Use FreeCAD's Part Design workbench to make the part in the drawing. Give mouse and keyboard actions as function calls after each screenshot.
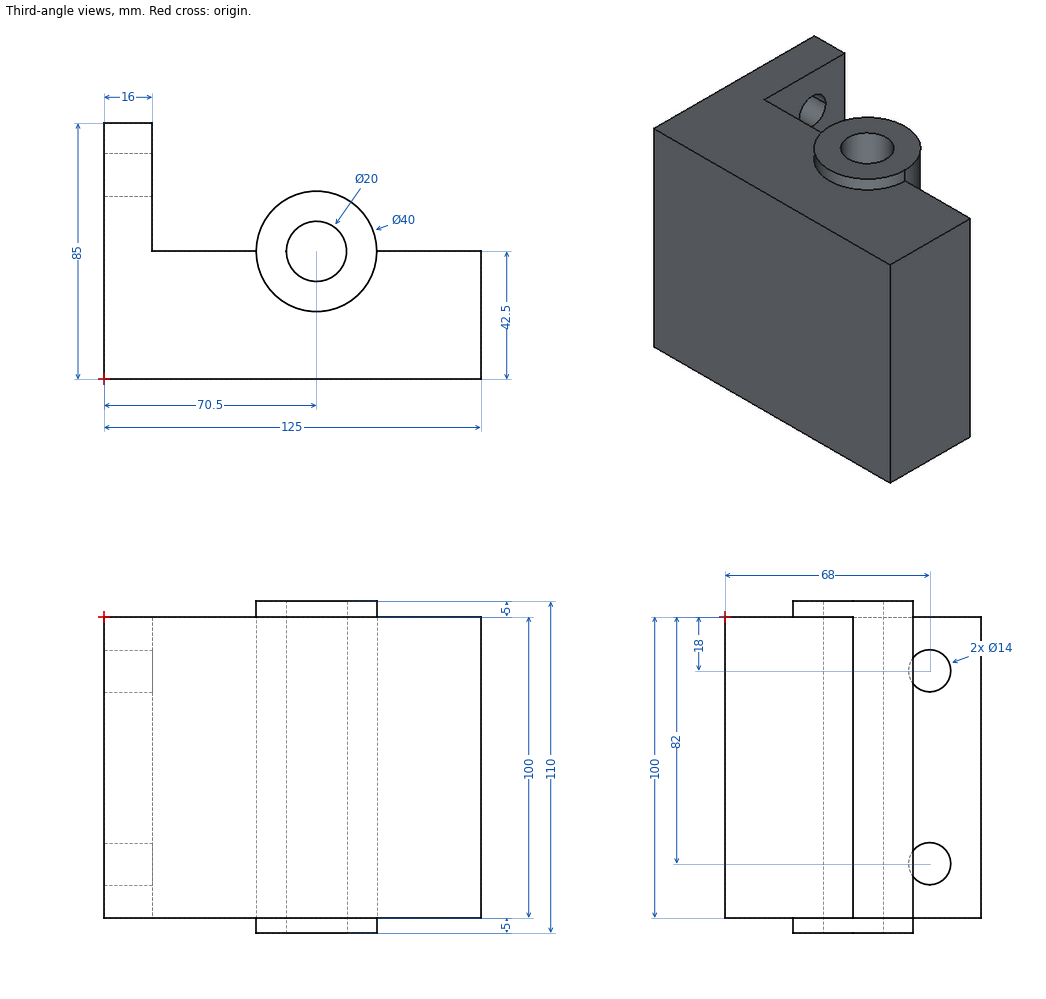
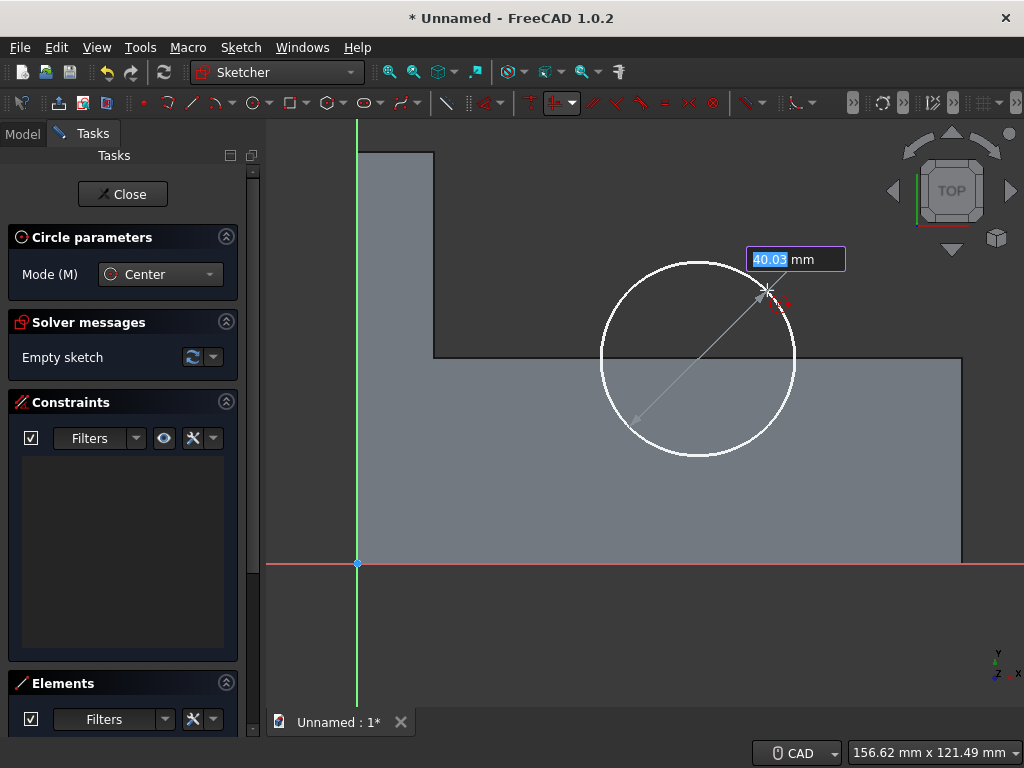
text(40)
key(Return)
key(Escape)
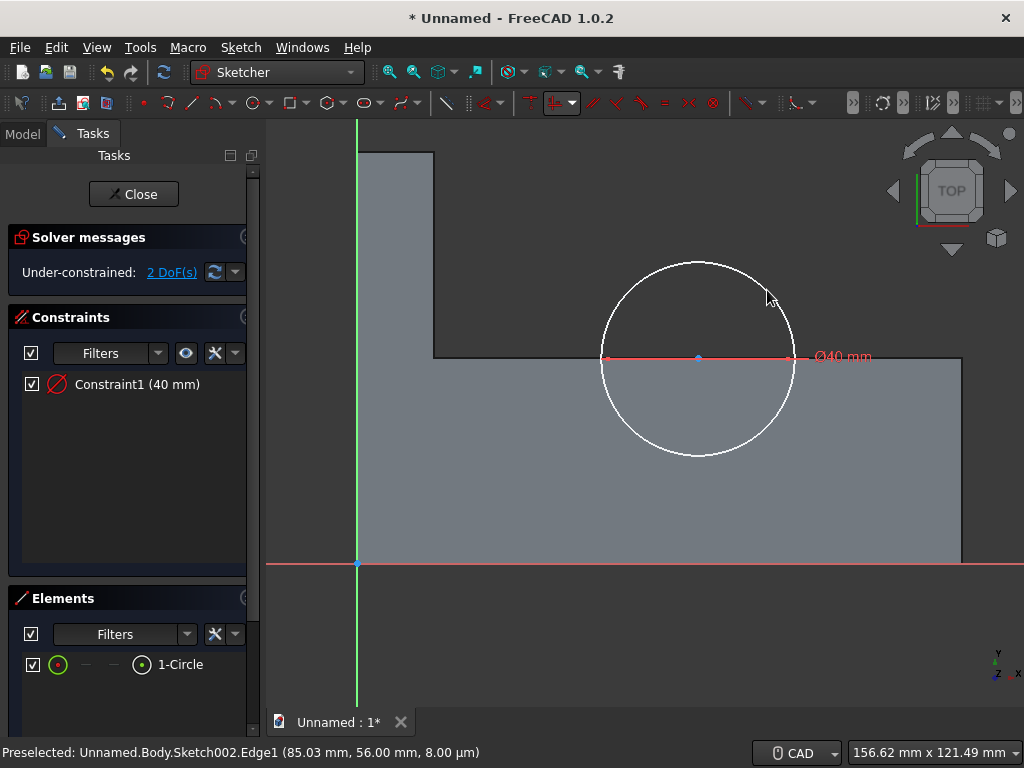
click(484, 104)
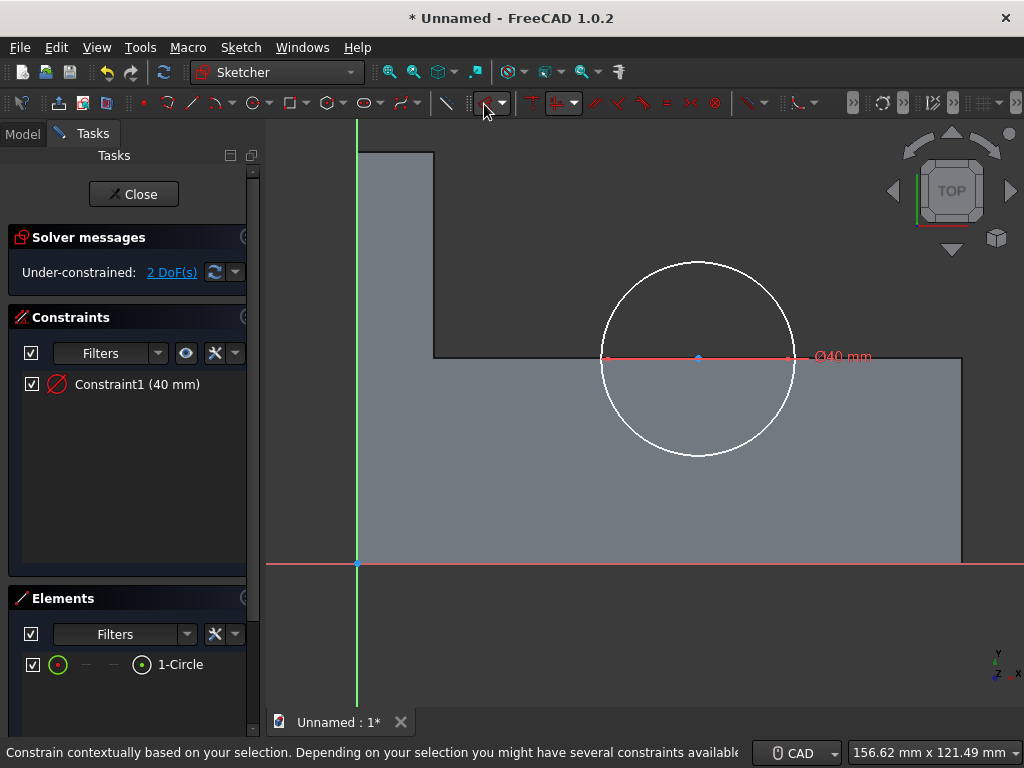
click(698, 359)
click(528, 598)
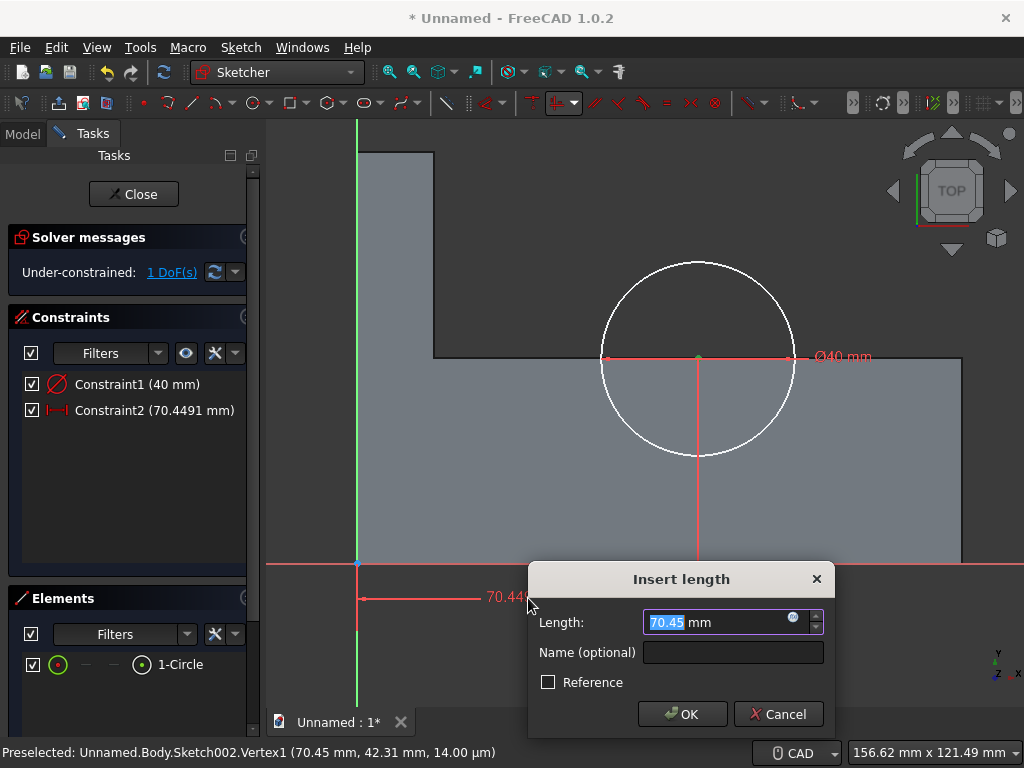
text(70.5)
key(Return)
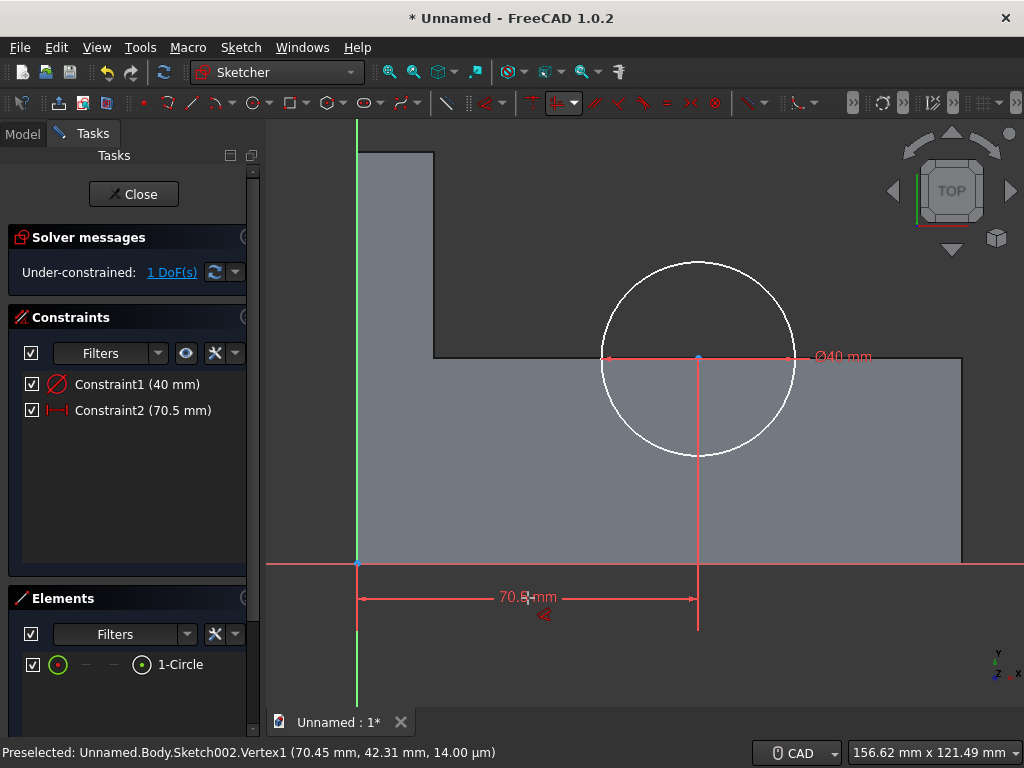
click(698, 359)
click(323, 461)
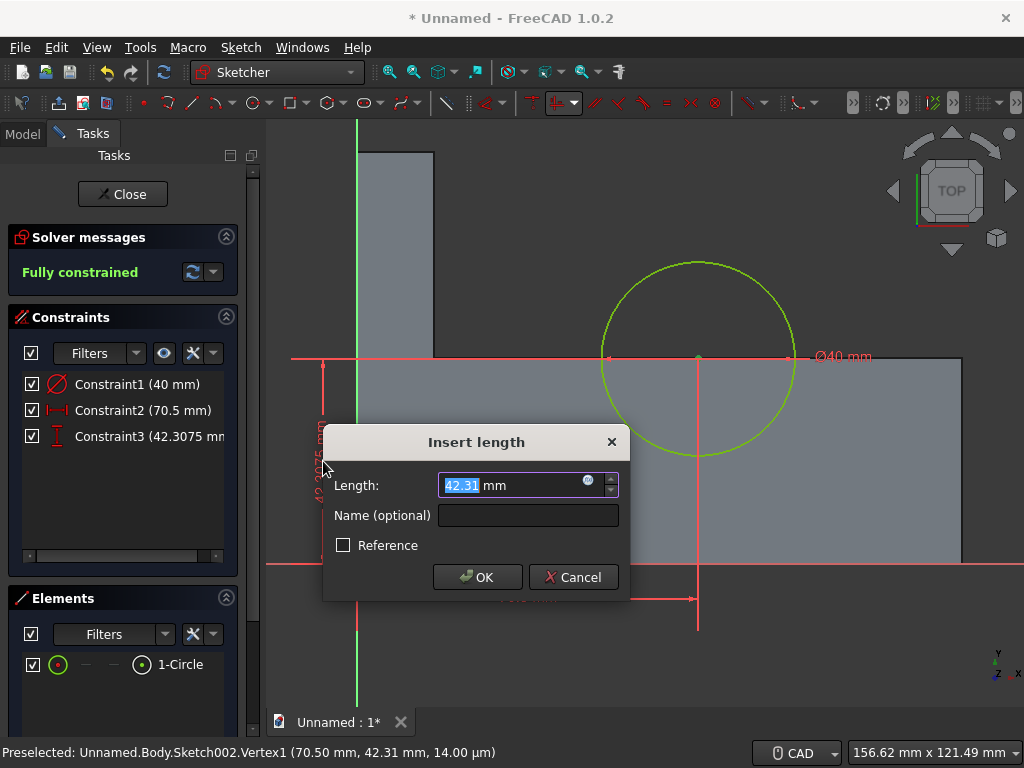
text(42.5)
key(Return)
key(Escape)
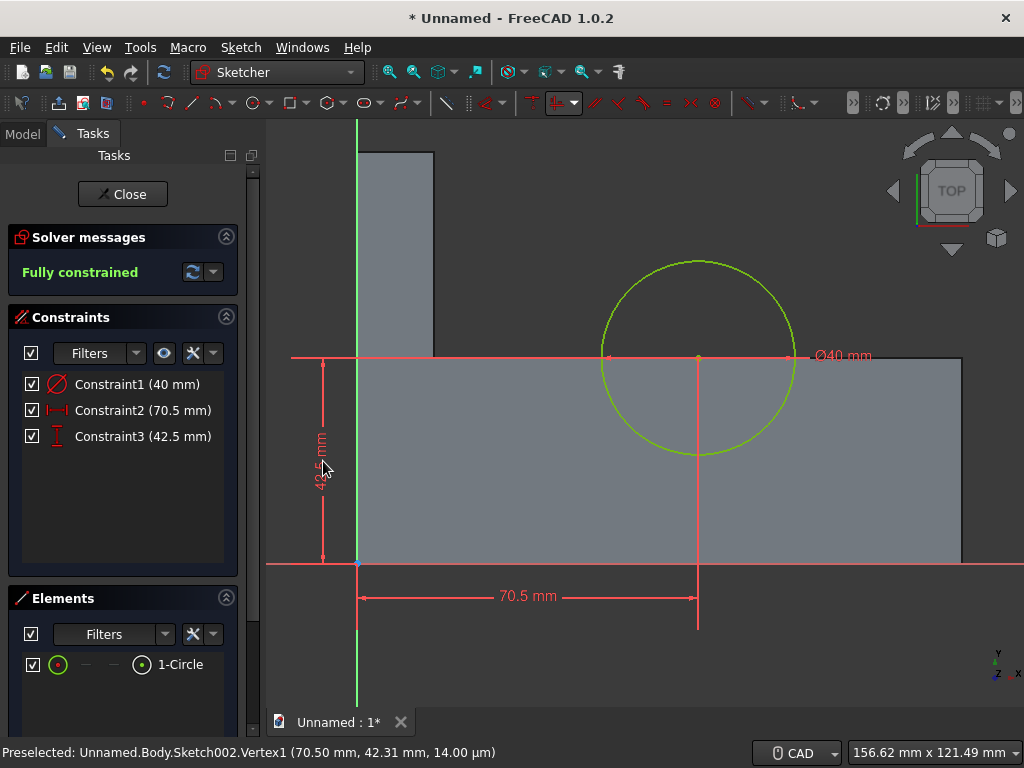
click(123, 194)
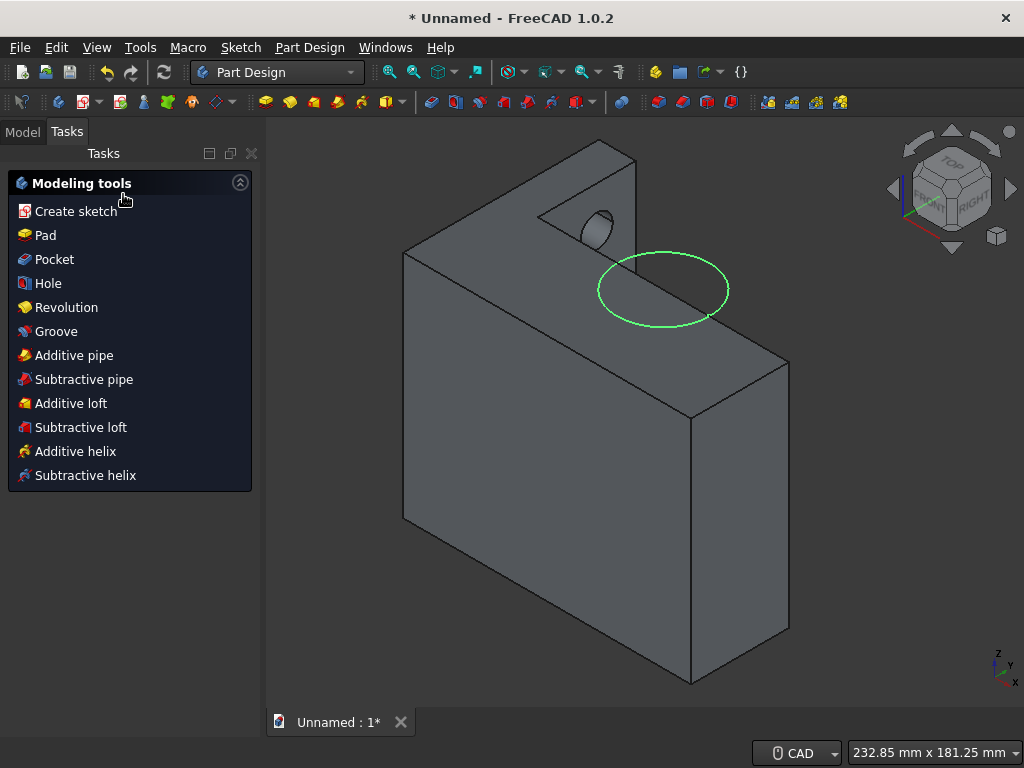
click(266, 102)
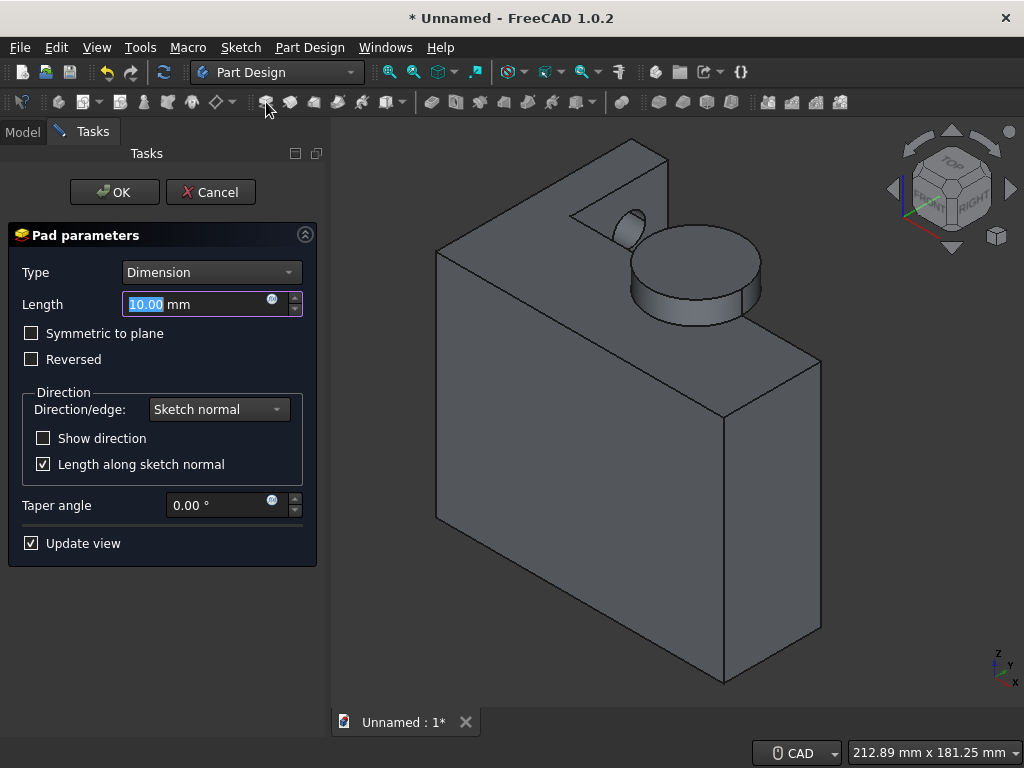
text(100)
key(Tab)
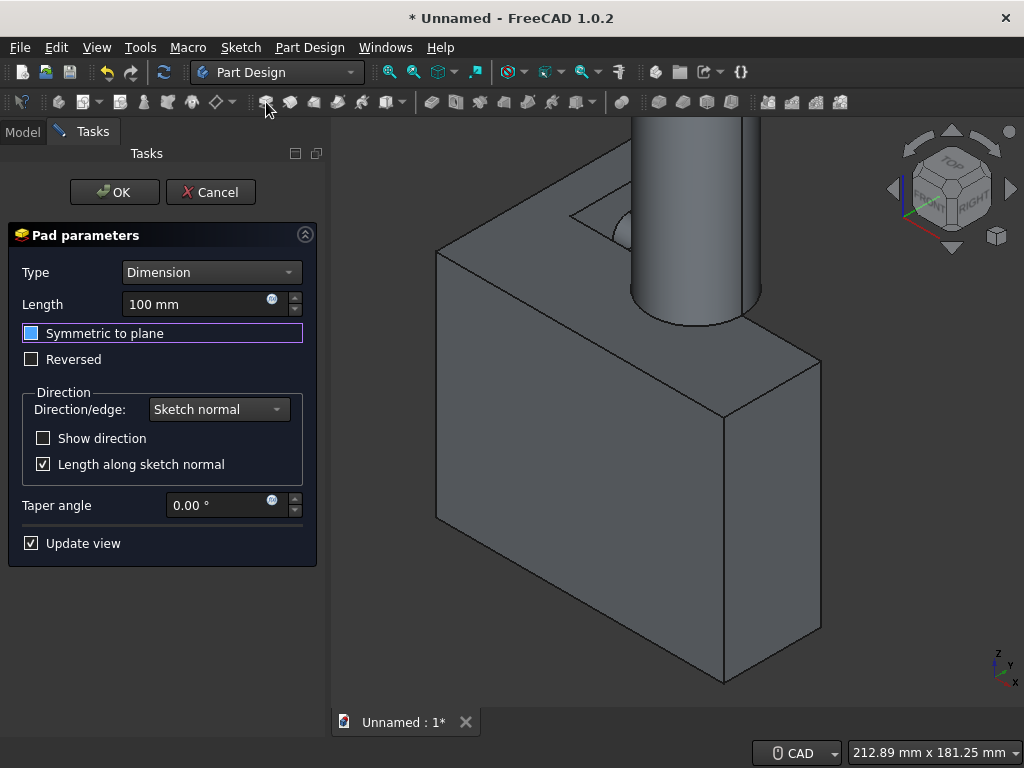
click(30, 359)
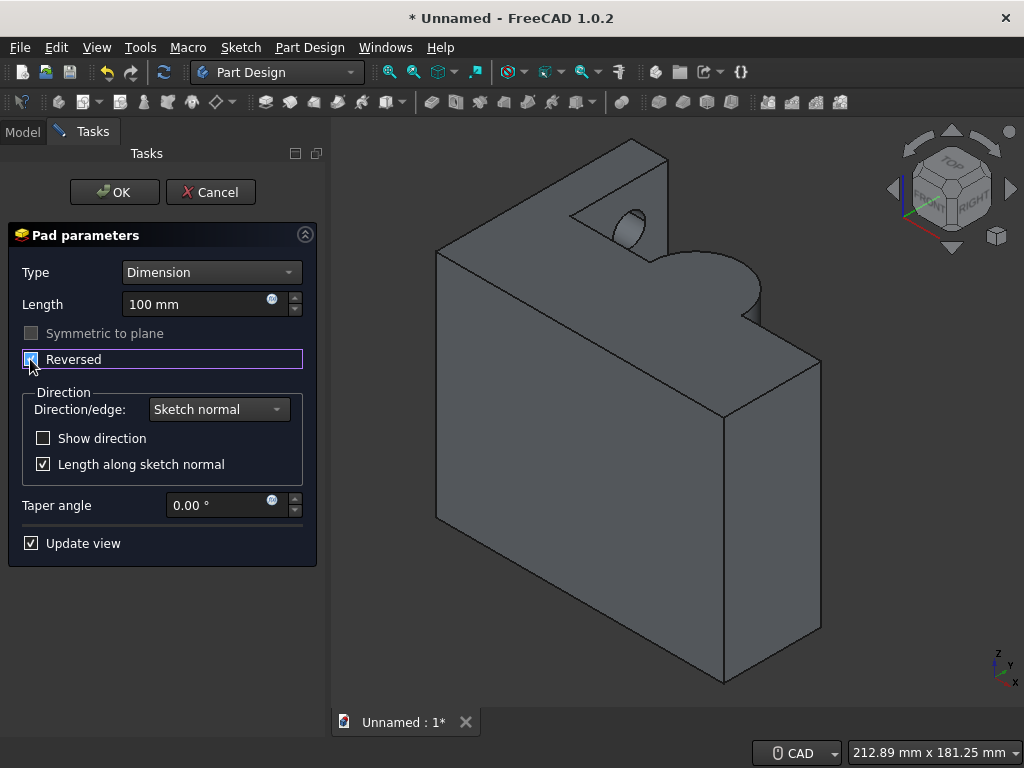
click(115, 192)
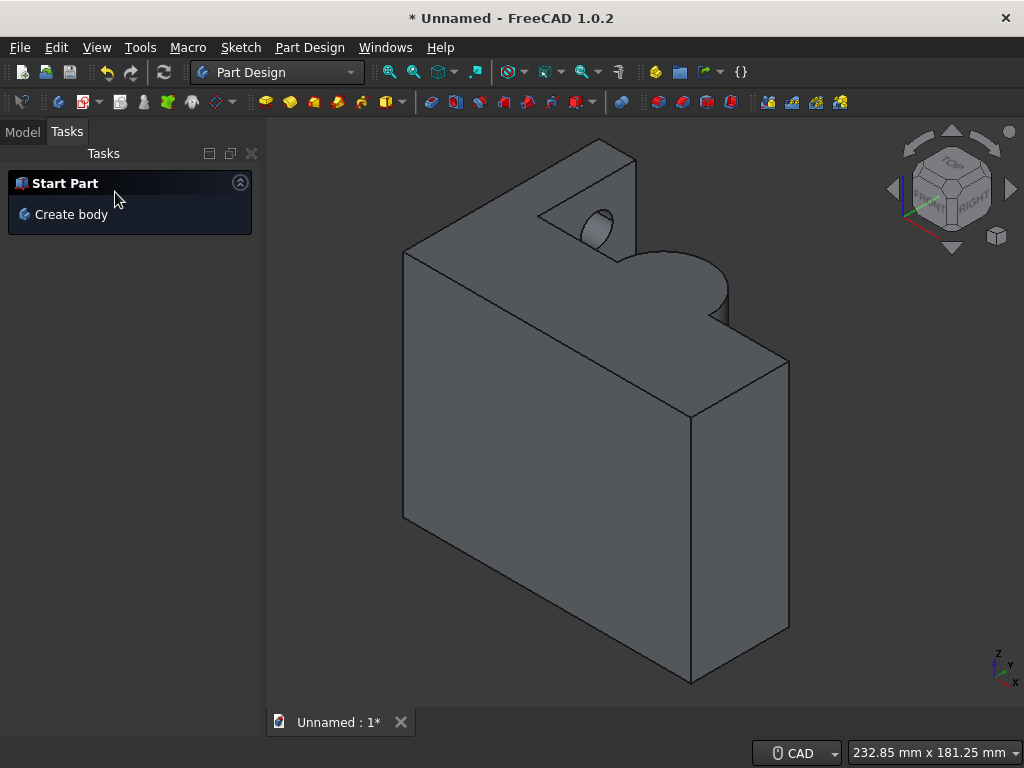
click(23, 131)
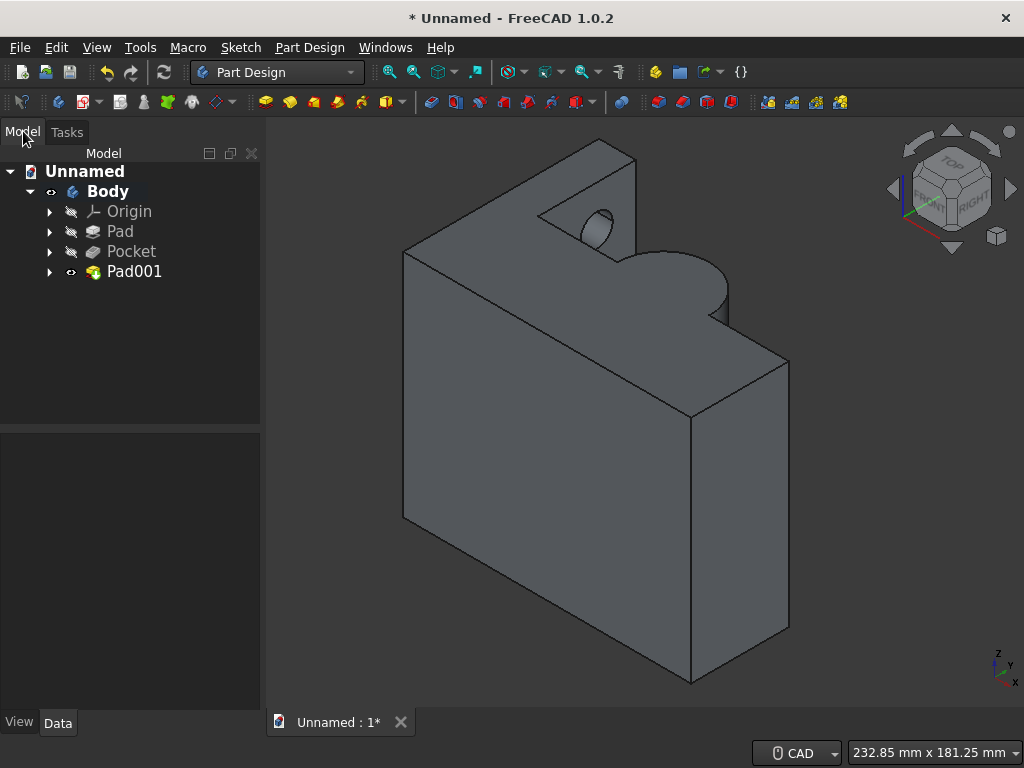
click(50, 212)